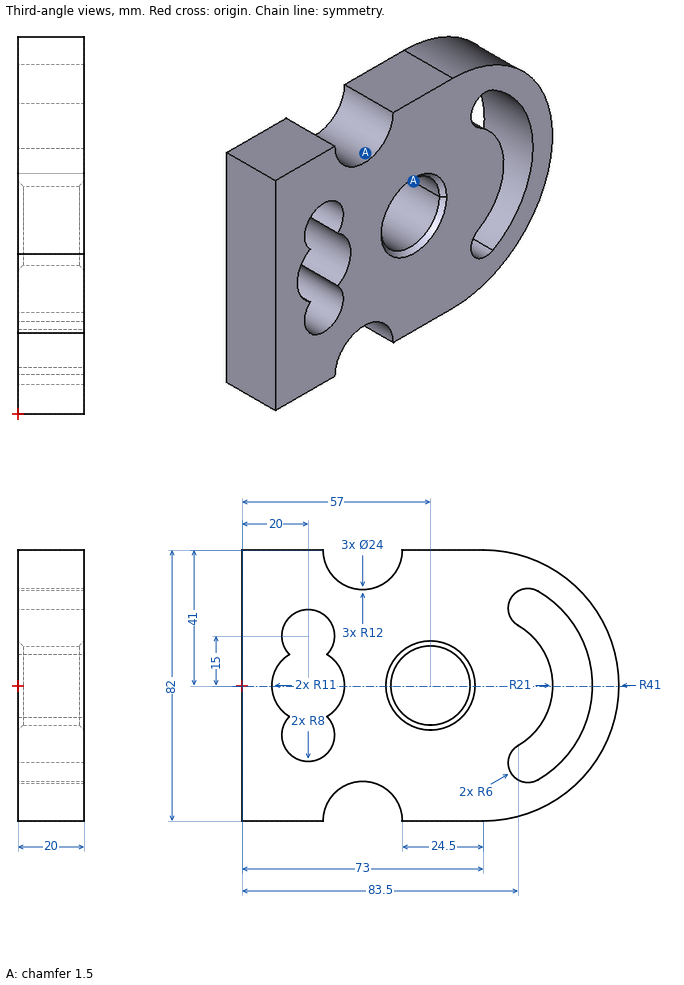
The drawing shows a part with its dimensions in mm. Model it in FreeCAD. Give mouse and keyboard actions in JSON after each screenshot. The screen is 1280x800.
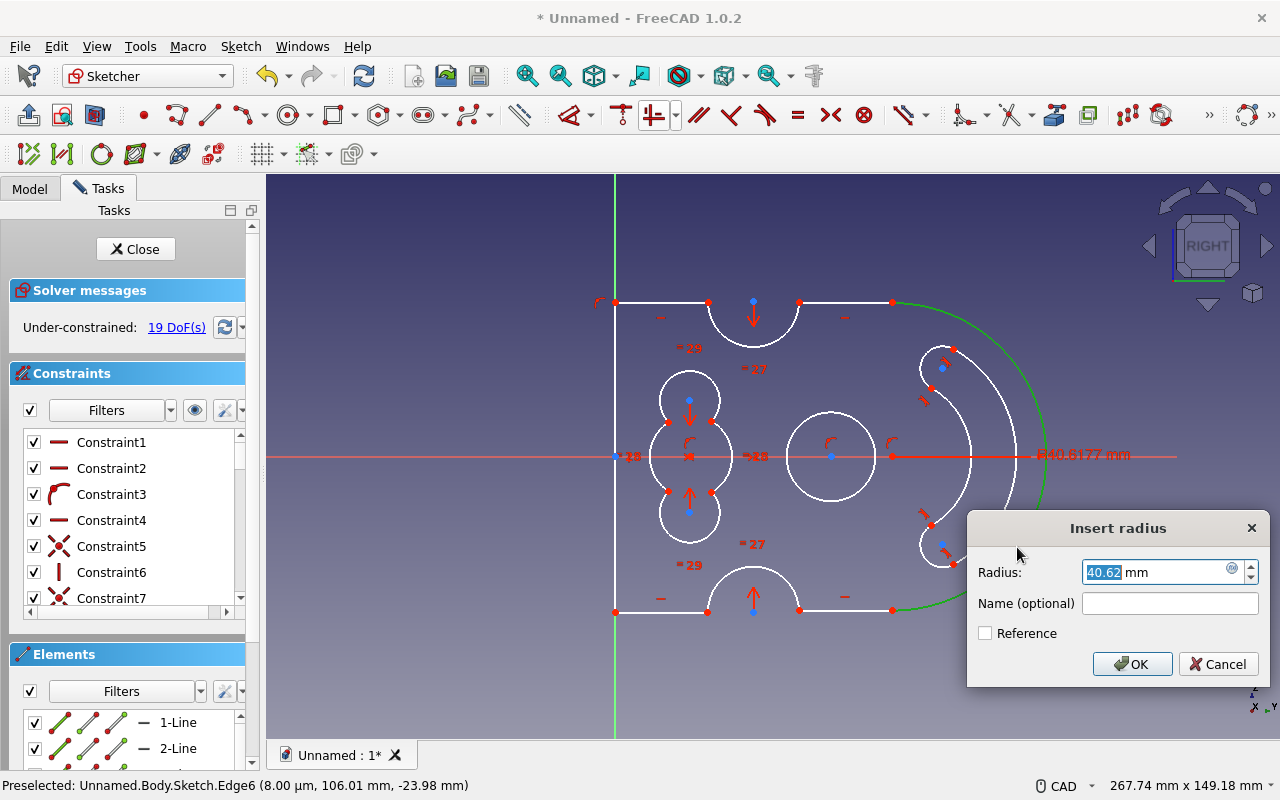
{"action": "type", "text": "41"}
{"action": "key", "text": "Return"}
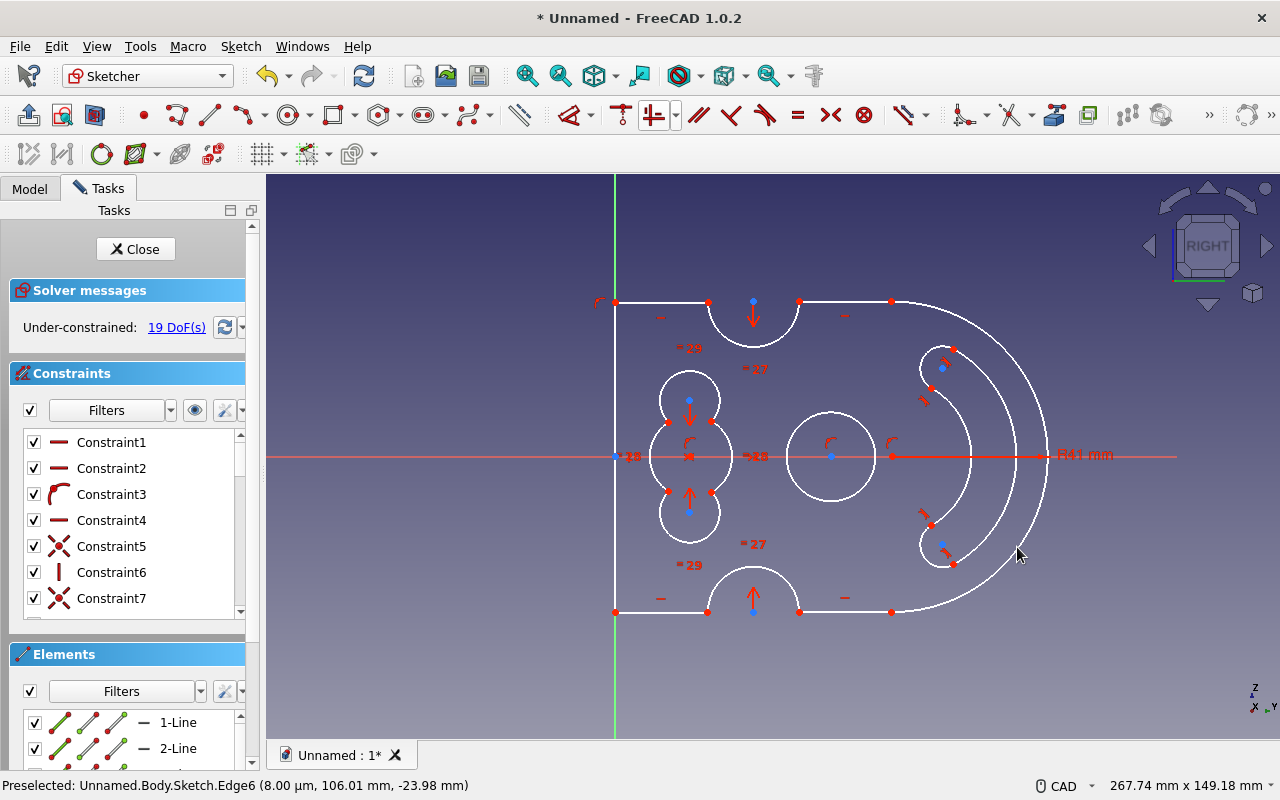
{"action": "left_click", "coordinate": [728, 339]}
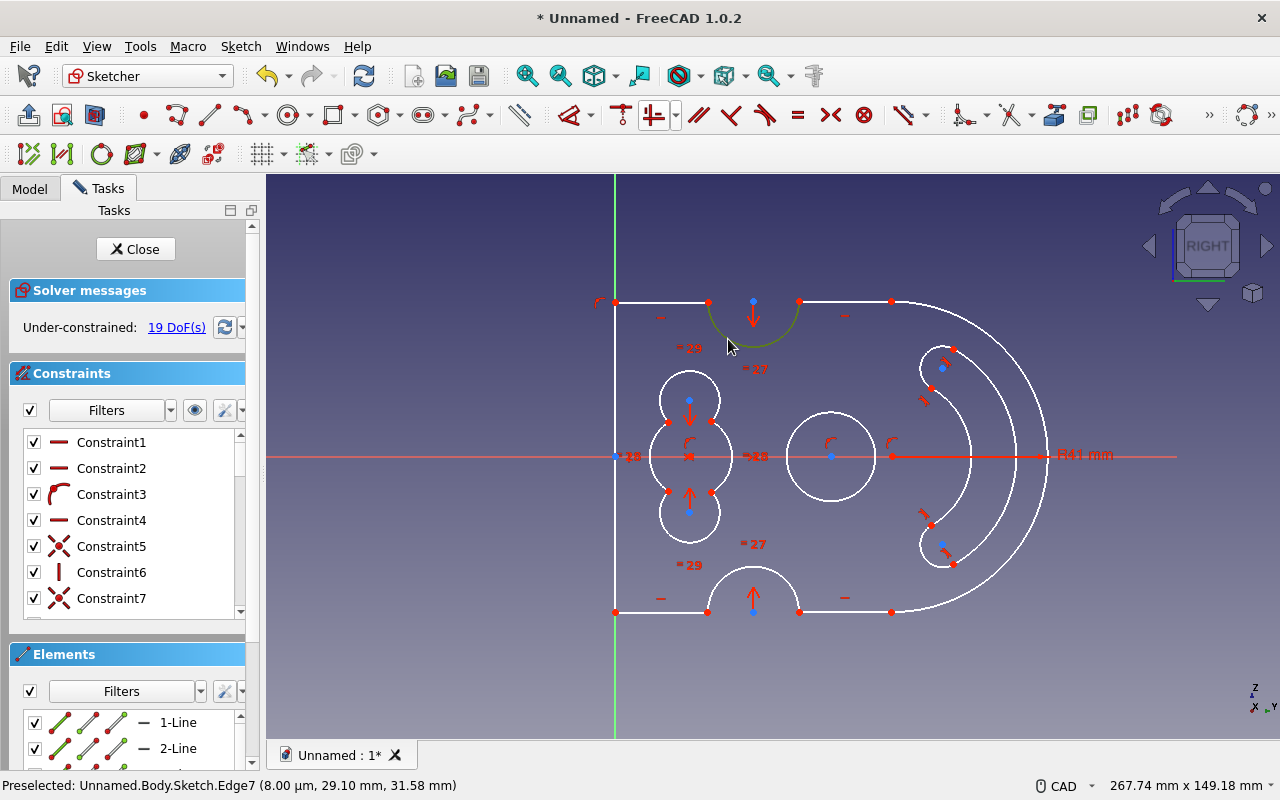
{"action": "key", "text": "k r"}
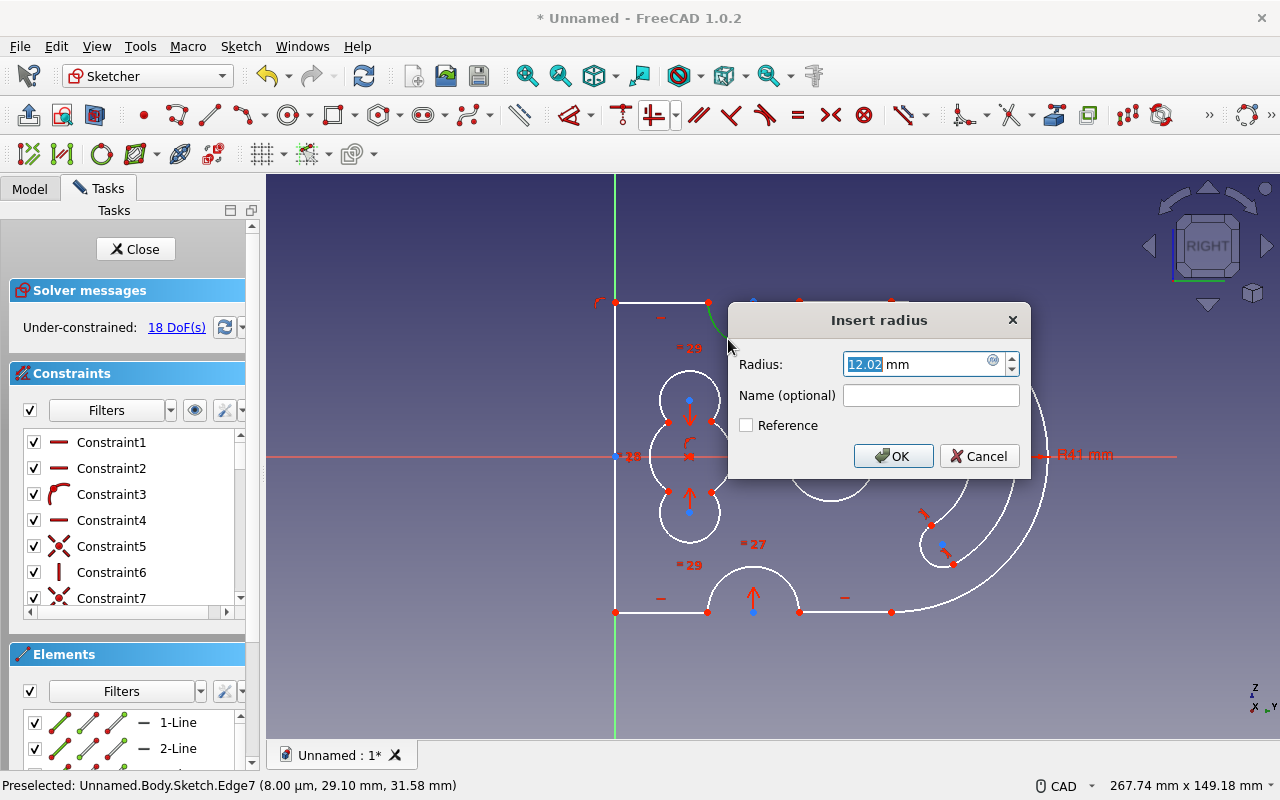
{"action": "type", "text": "12"}
{"action": "key", "text": "Return"}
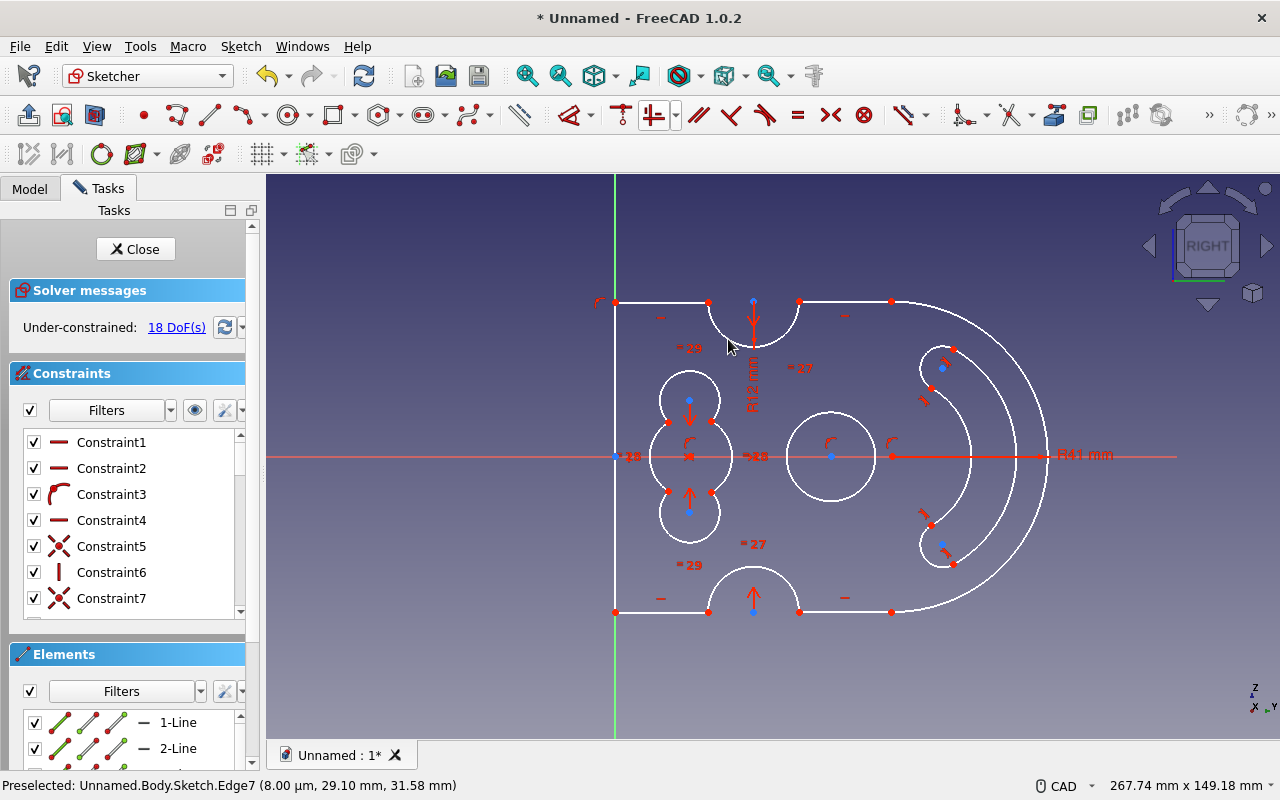
{"action": "left_click", "coordinate": [653, 441]}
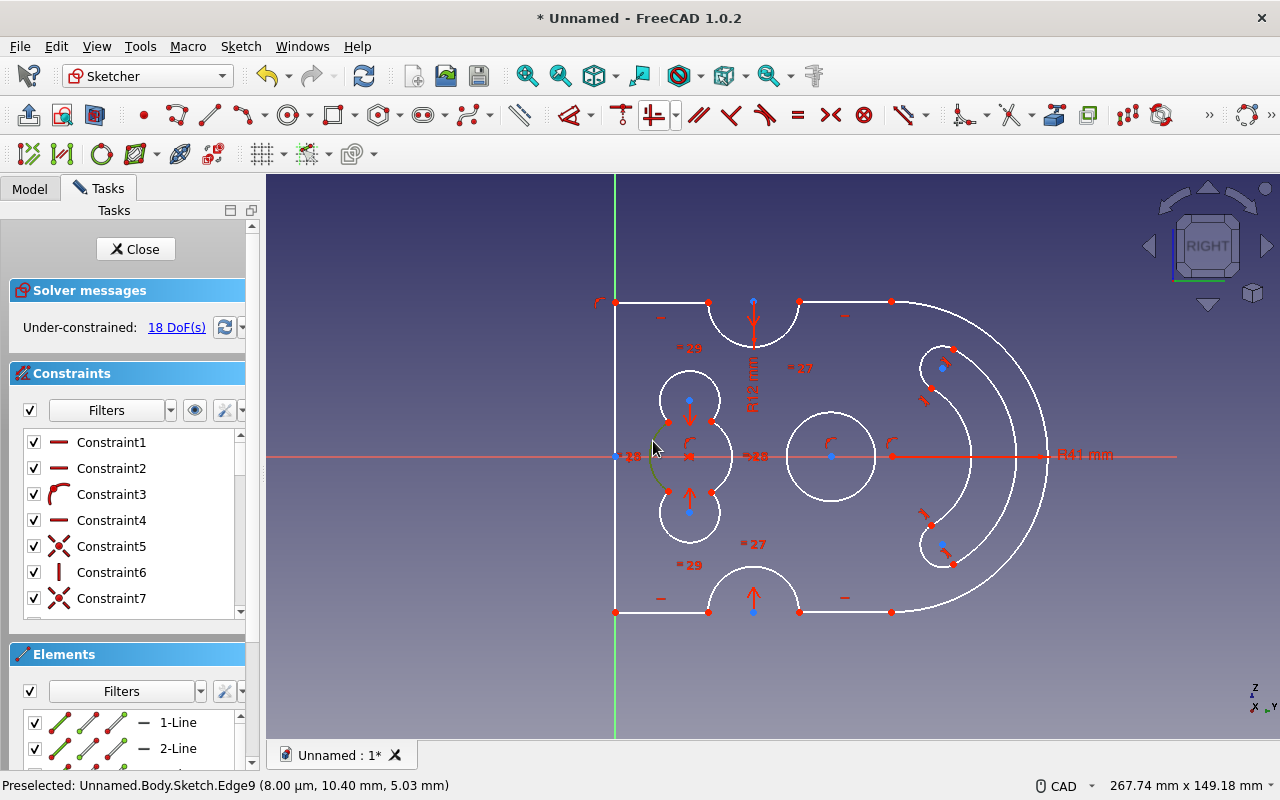
{"action": "left_click", "coordinate": [590, 116]}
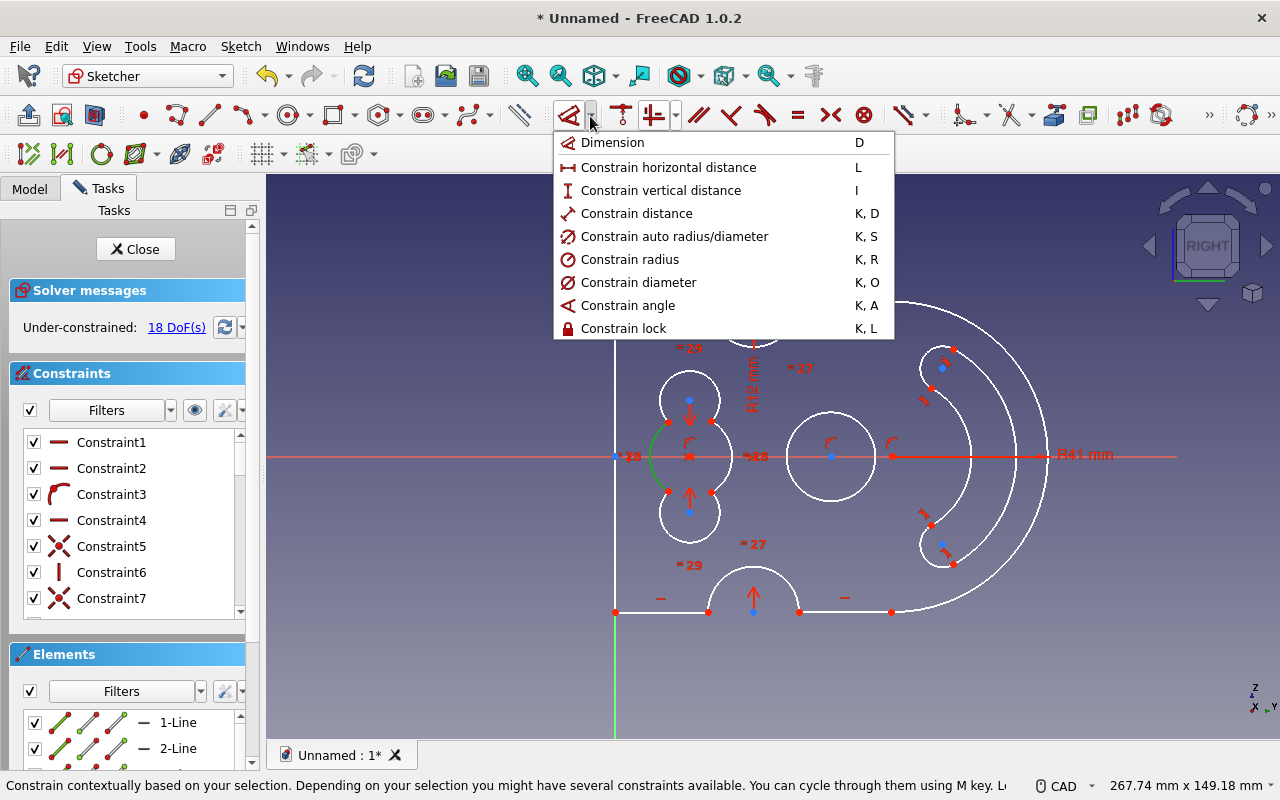
{"action": "left_click", "coordinate": [724, 260]}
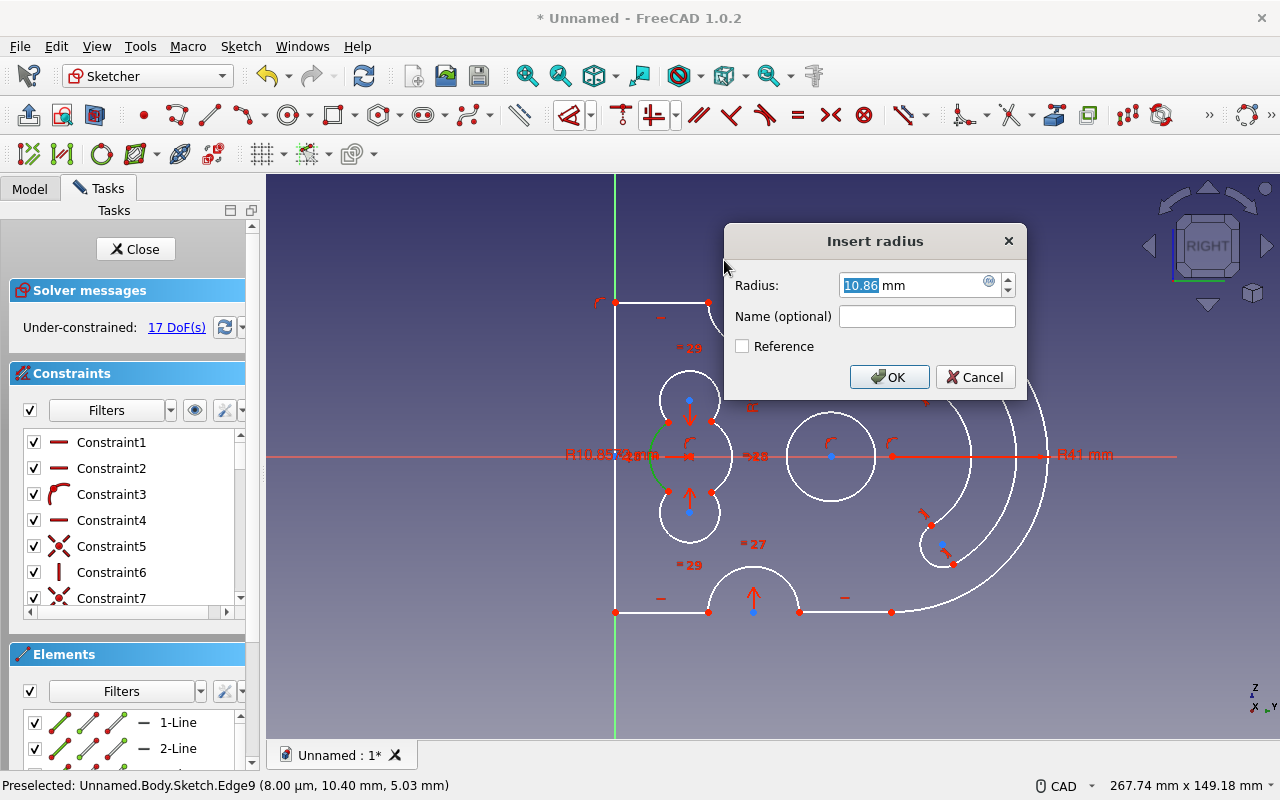
{"action": "type", "text": "11"}
{"action": "key", "text": "Return"}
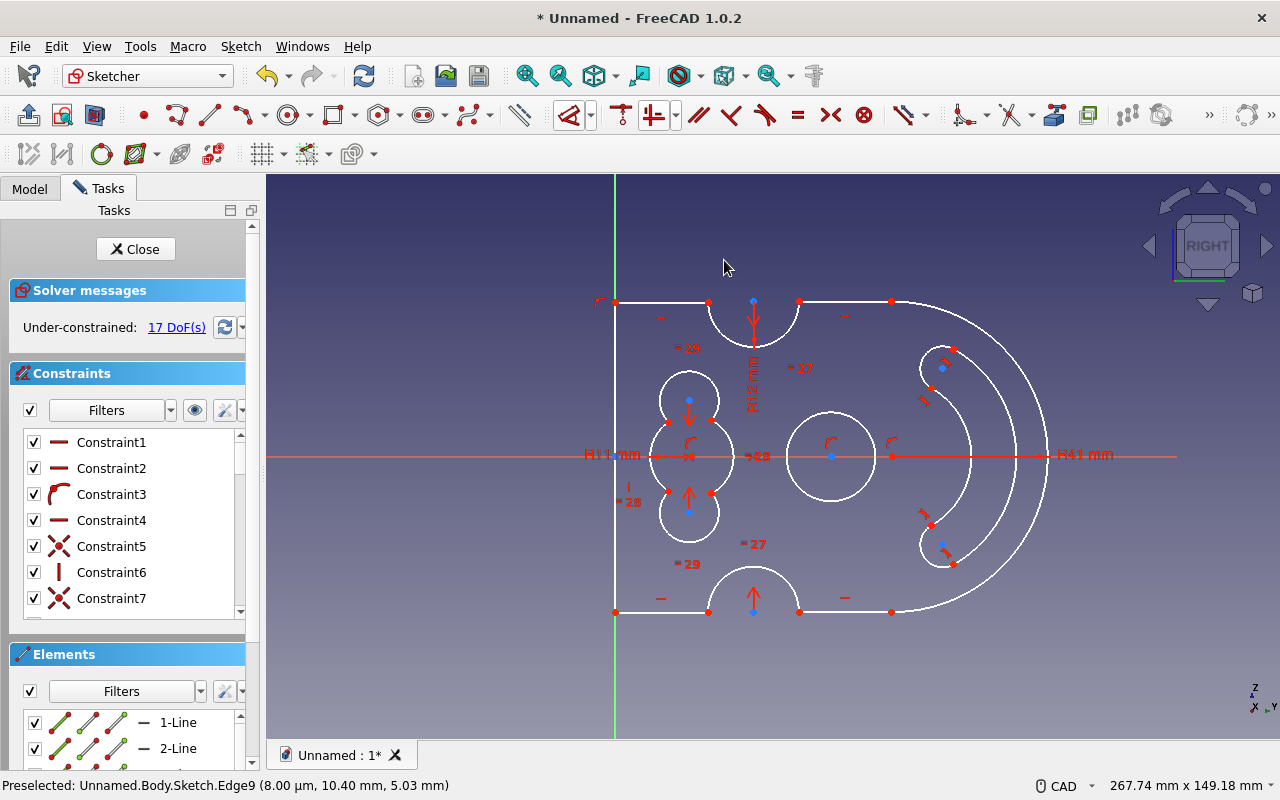
{"action": "scroll", "coordinate": [712, 382], "scroll_direction": "up", "scroll_amount": 2}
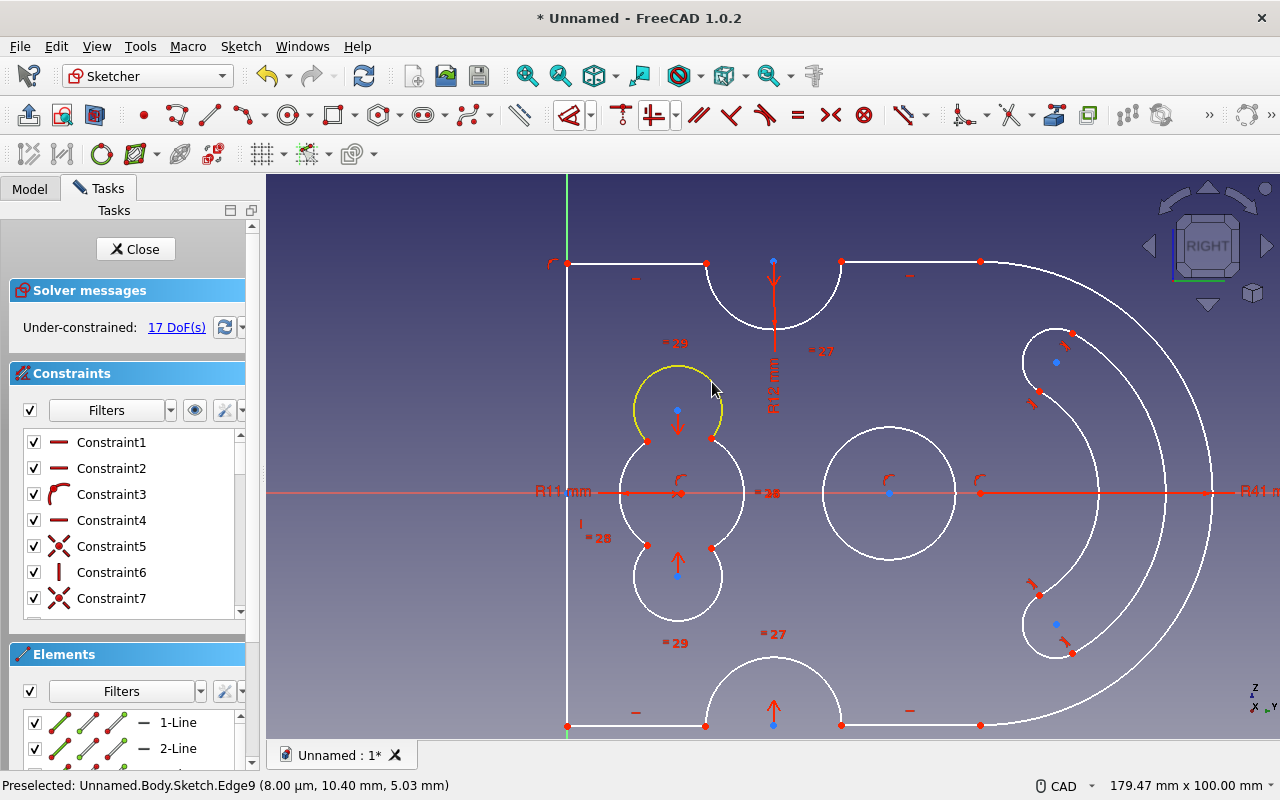
{"action": "left_click", "coordinate": [712, 382]}